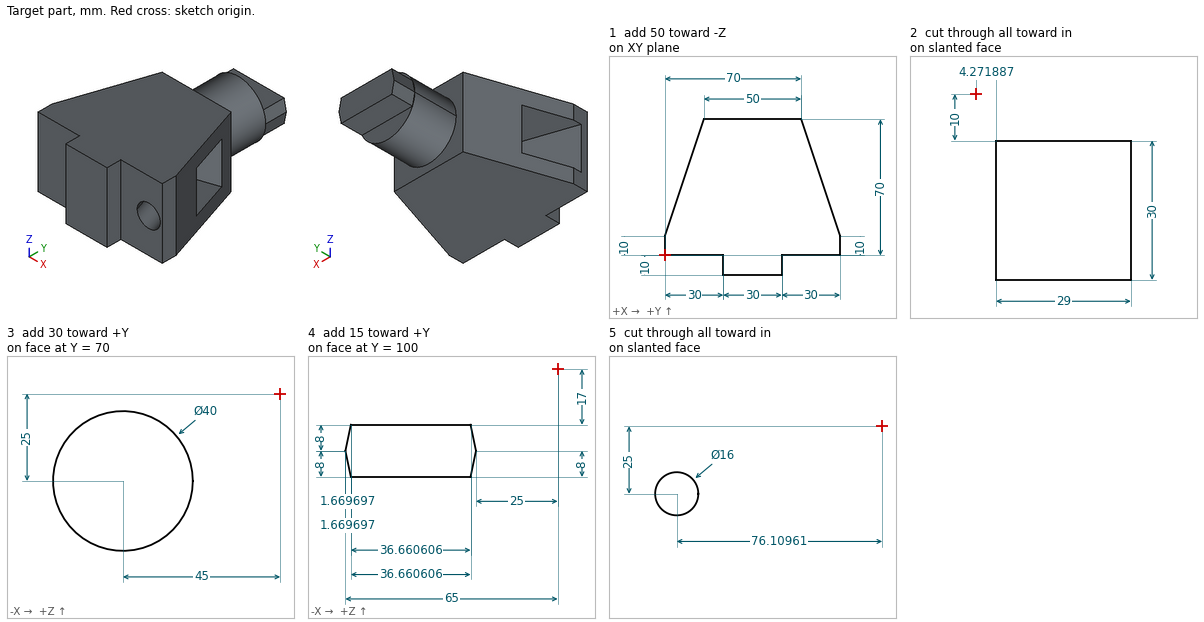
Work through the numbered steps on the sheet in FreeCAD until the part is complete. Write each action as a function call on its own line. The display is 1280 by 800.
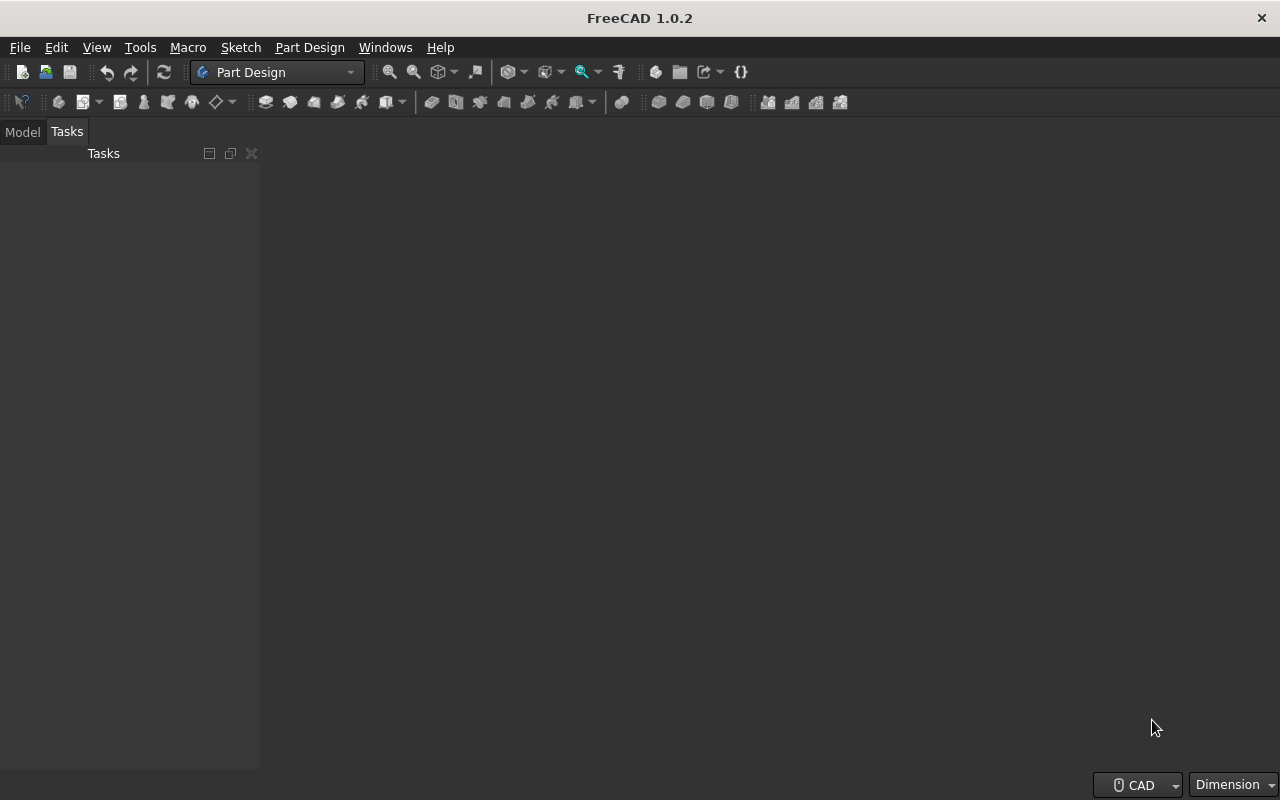
key(ctrl+n)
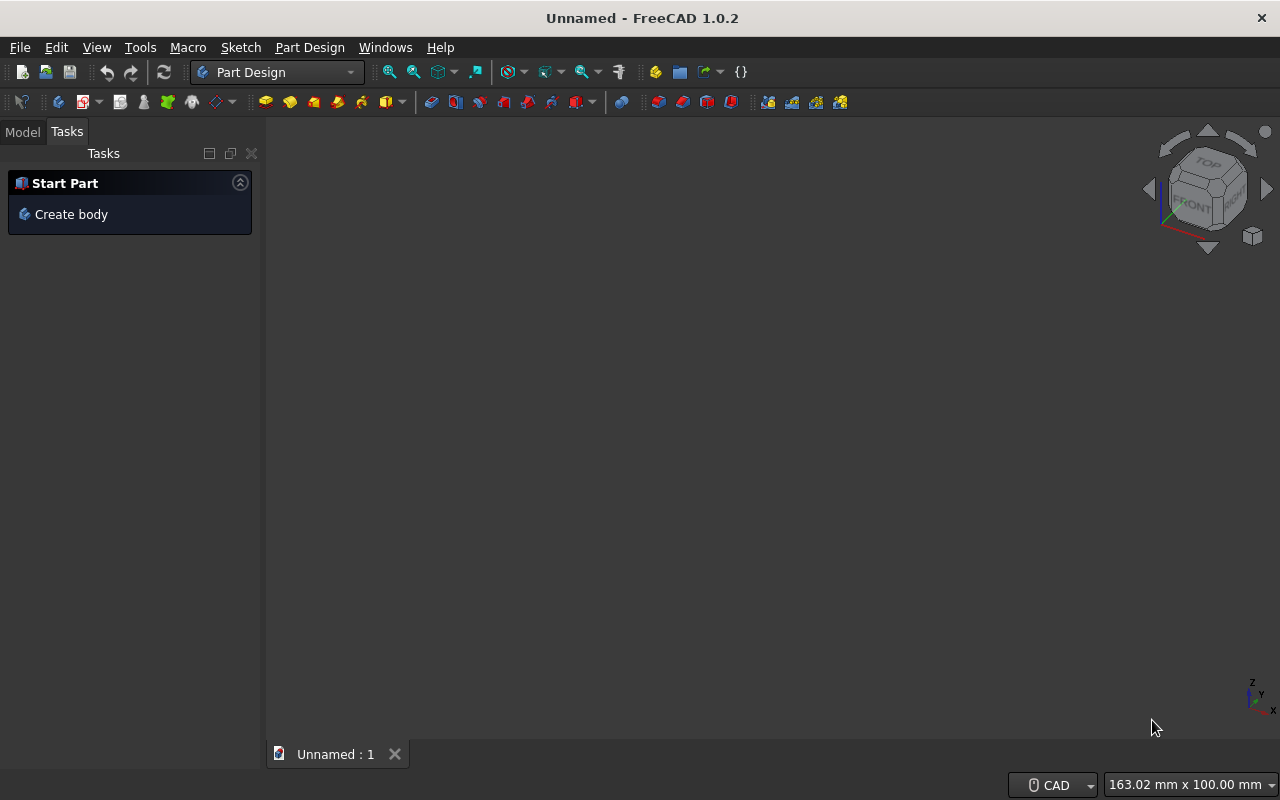
click(84, 102)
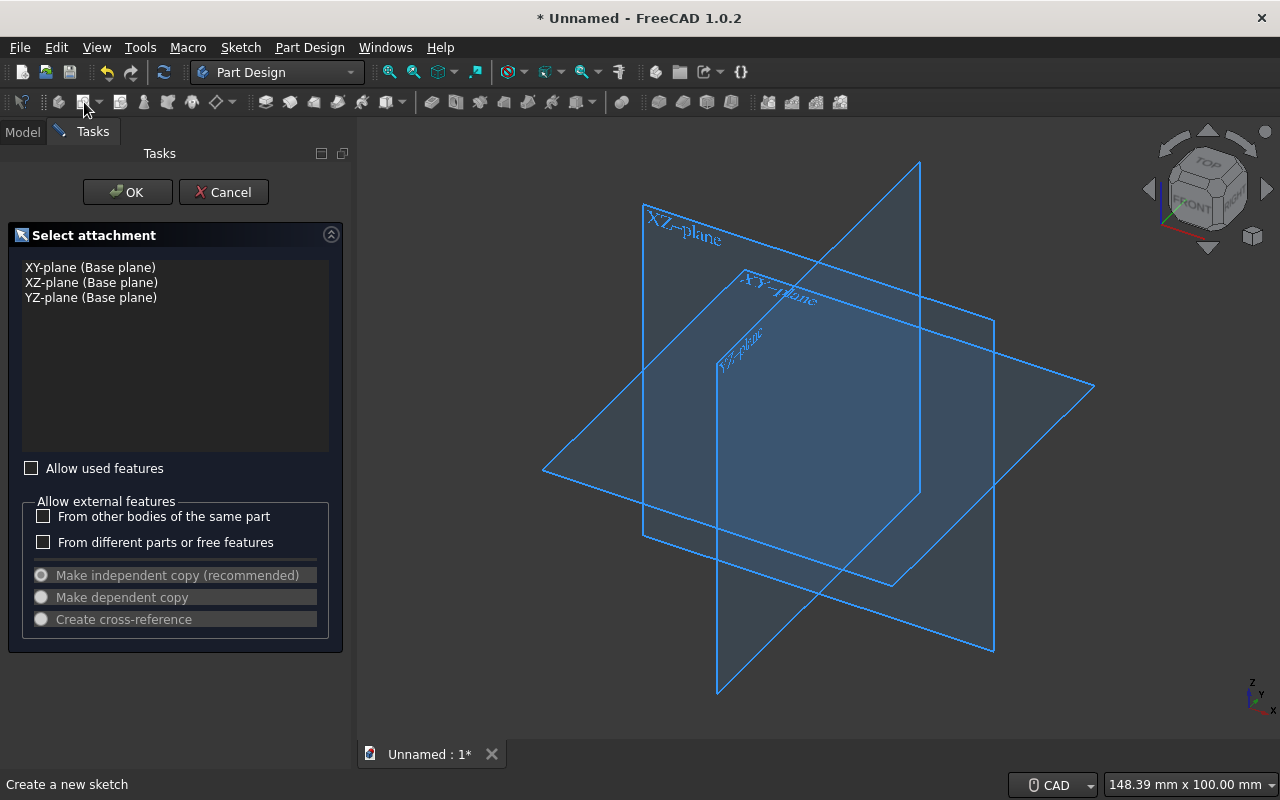
click(82, 268)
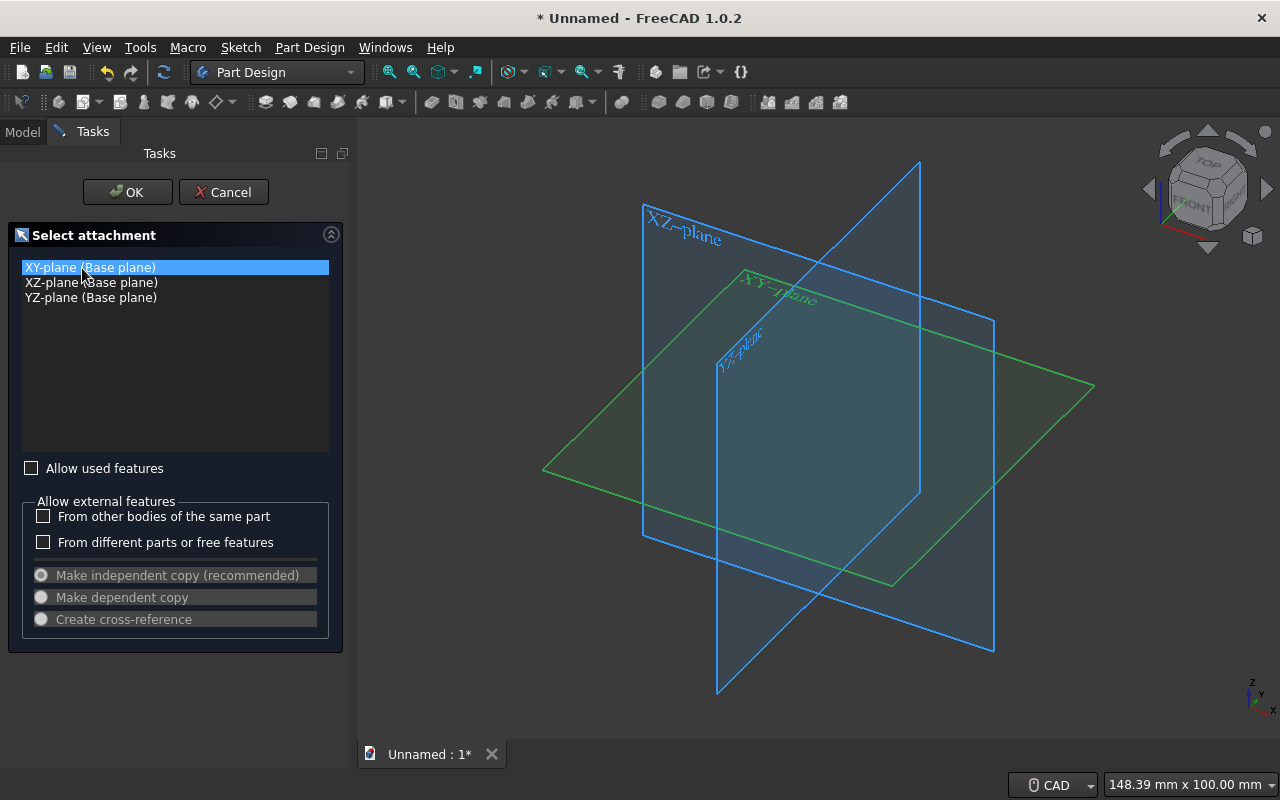
click(128, 192)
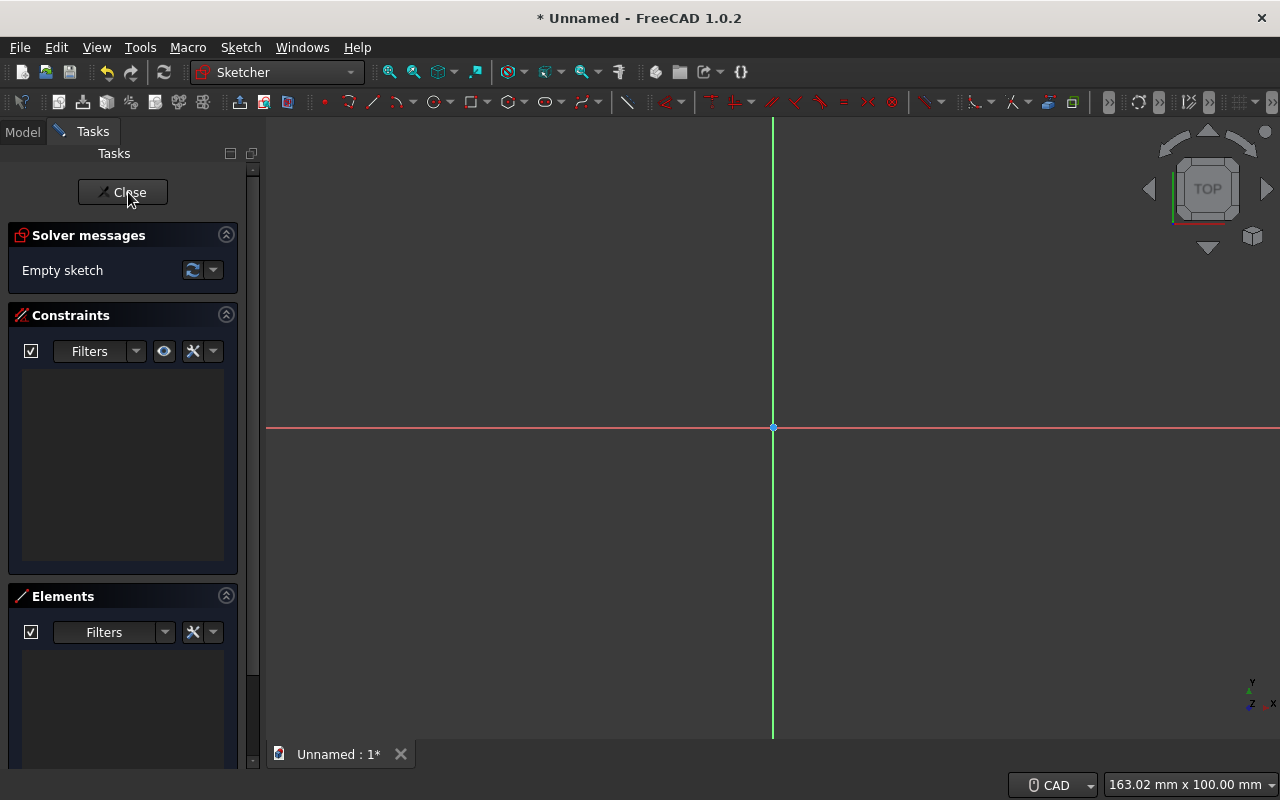
scroll(294, 711, down, 2)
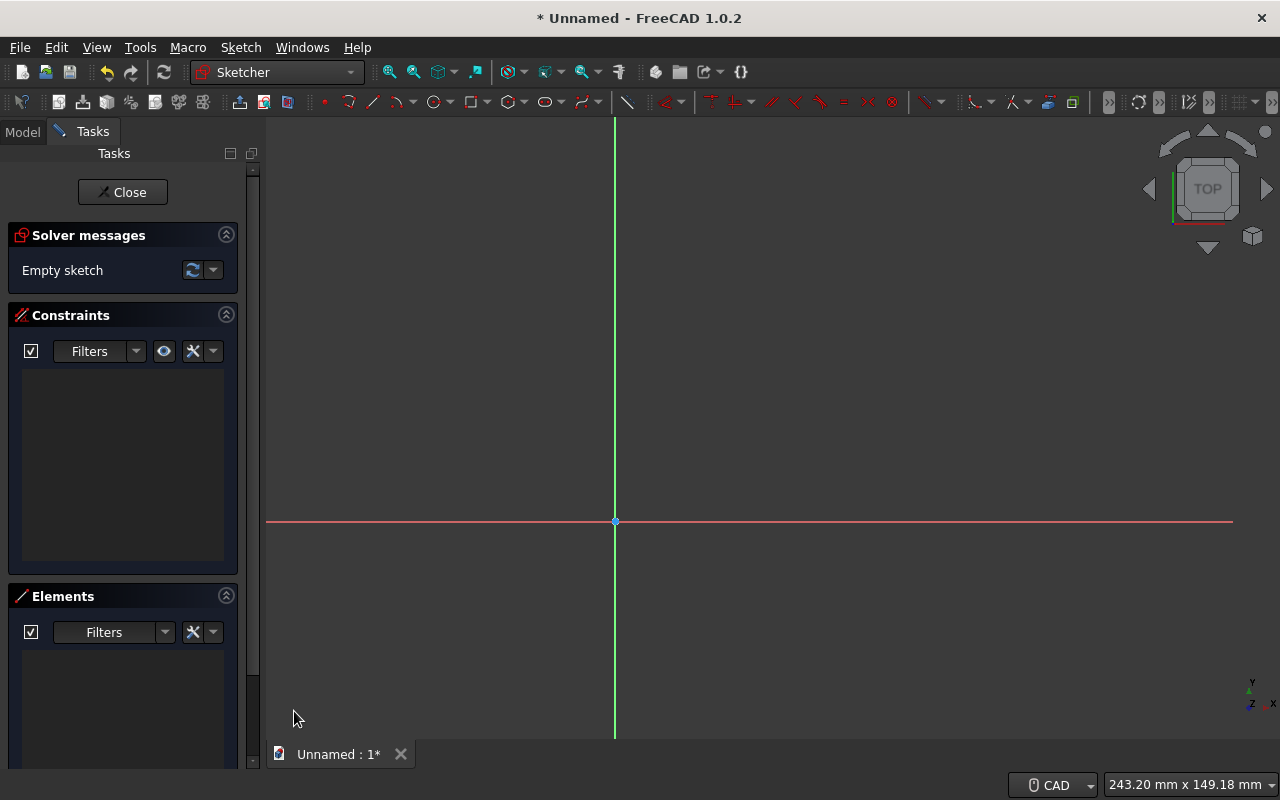
click(350, 102)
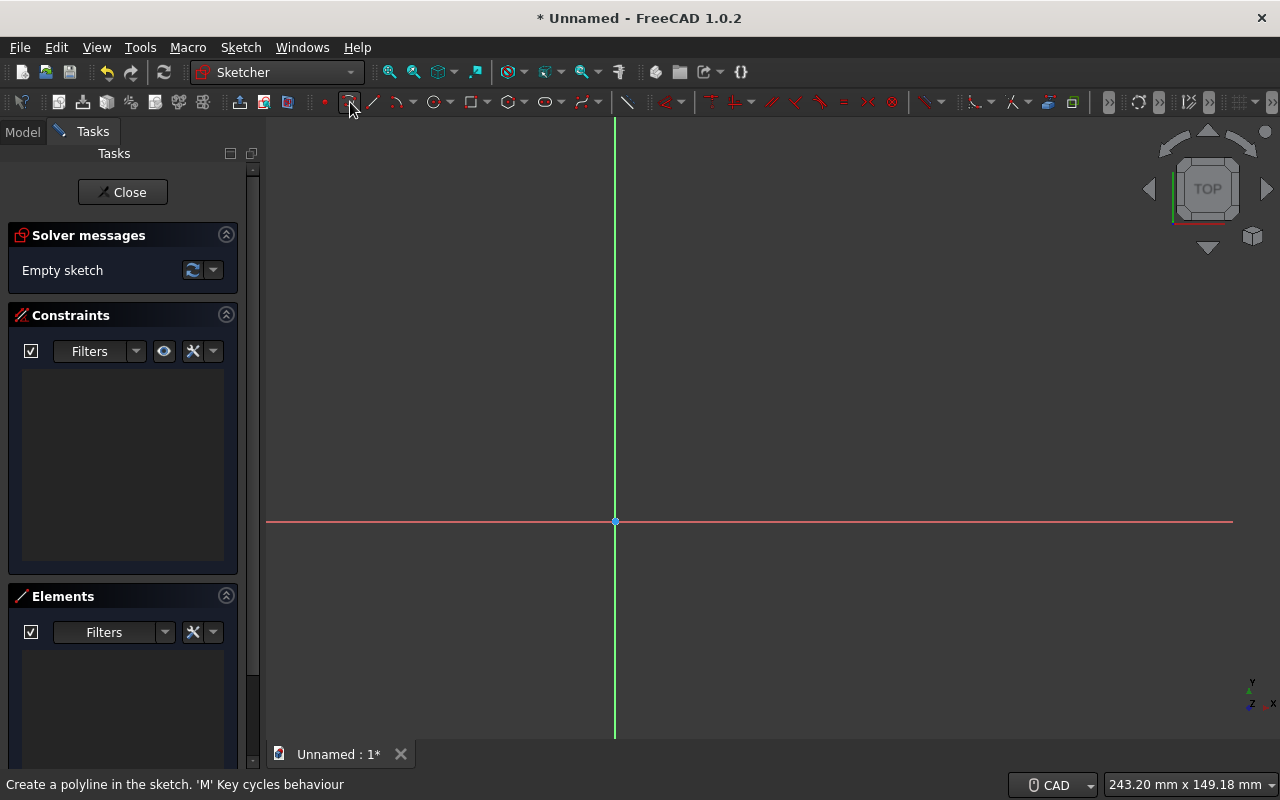
click(615, 522)
click(740, 513)
click(740, 563)
click(865, 563)
click(865, 522)
click(990, 513)
click(990, 480)
click(907, 230)
click(698, 230)
click(624, 480)
click(615, 522)
key(Escape)
key(Escape)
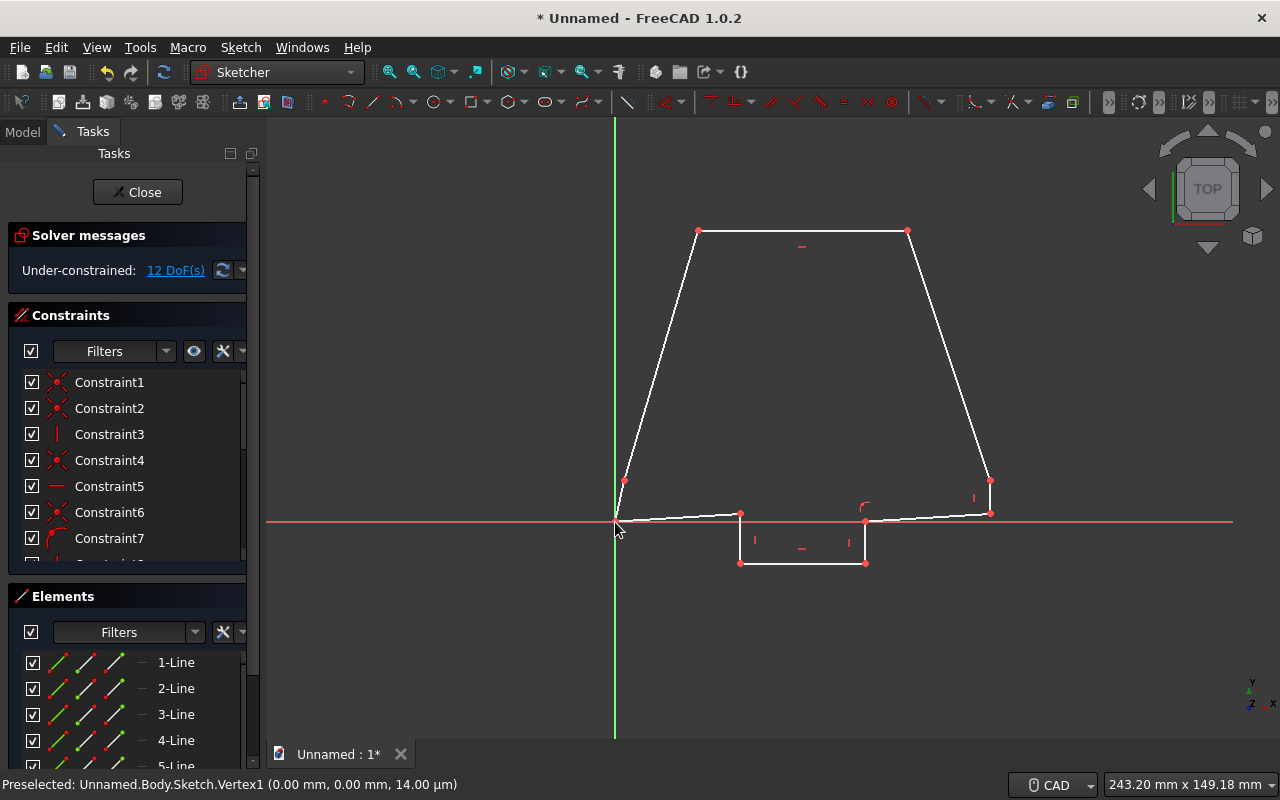
click(653, 519)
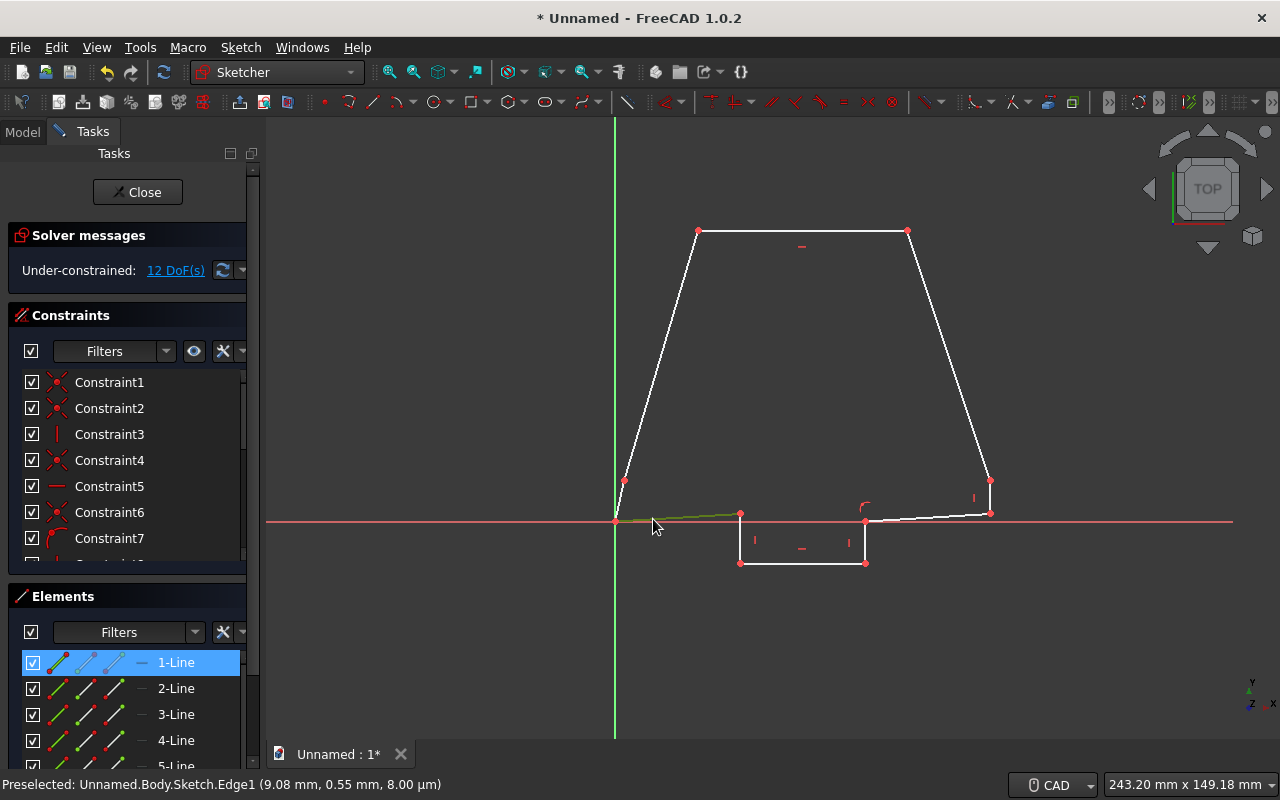
key(h)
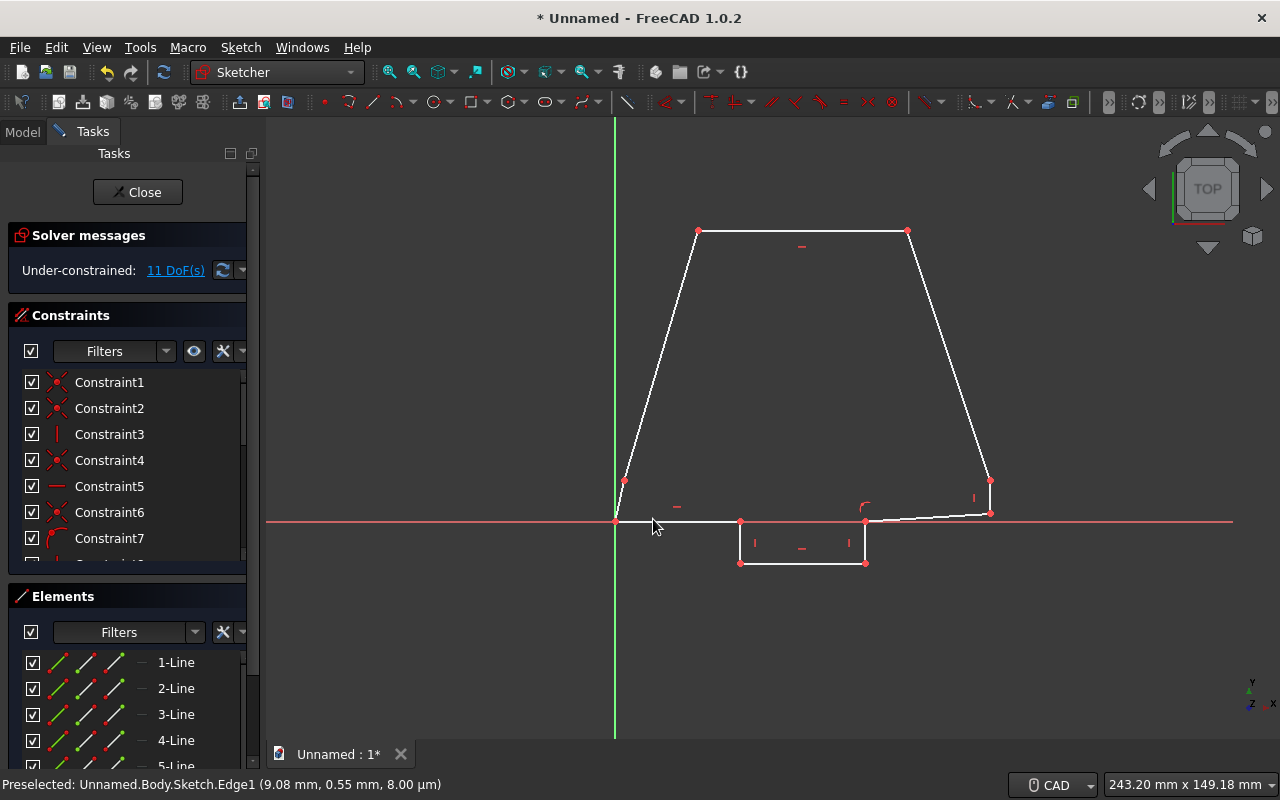
click(902, 519)